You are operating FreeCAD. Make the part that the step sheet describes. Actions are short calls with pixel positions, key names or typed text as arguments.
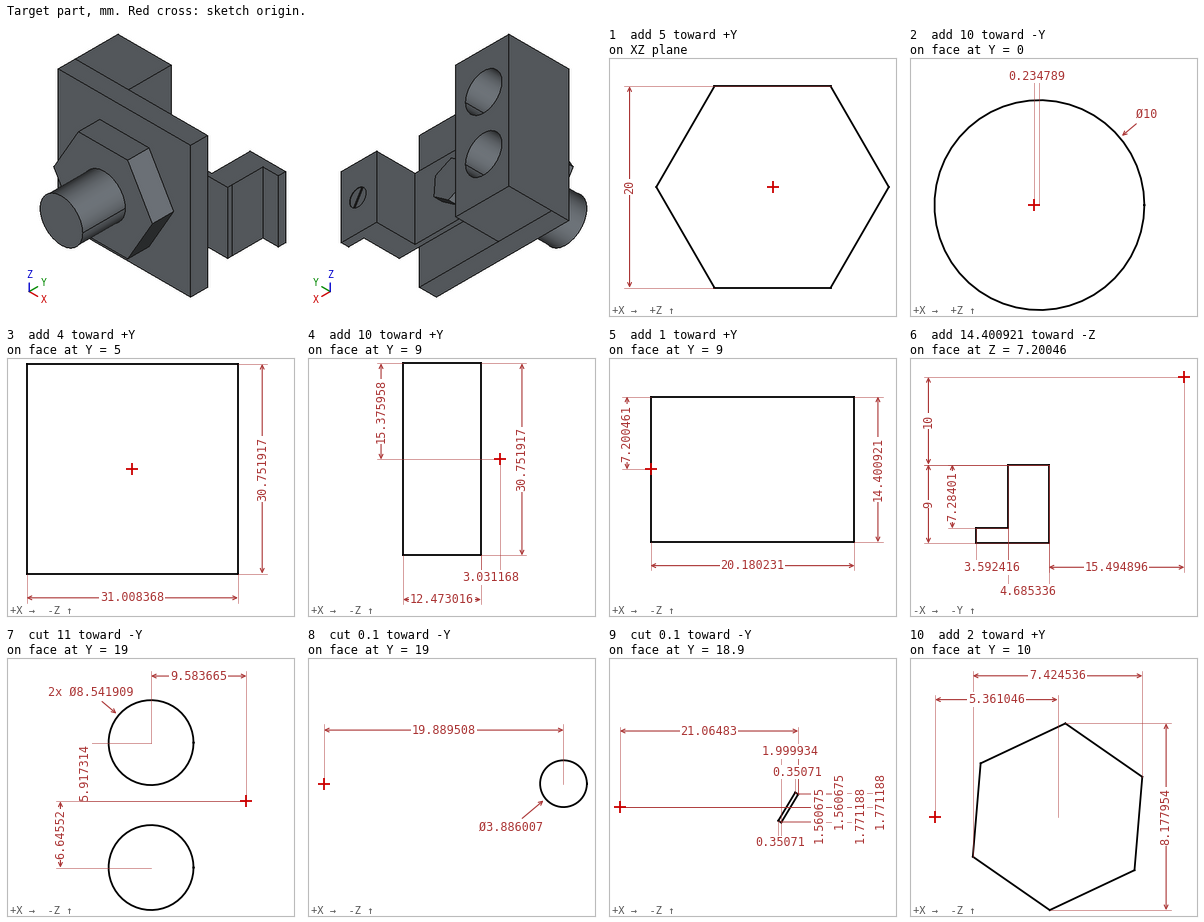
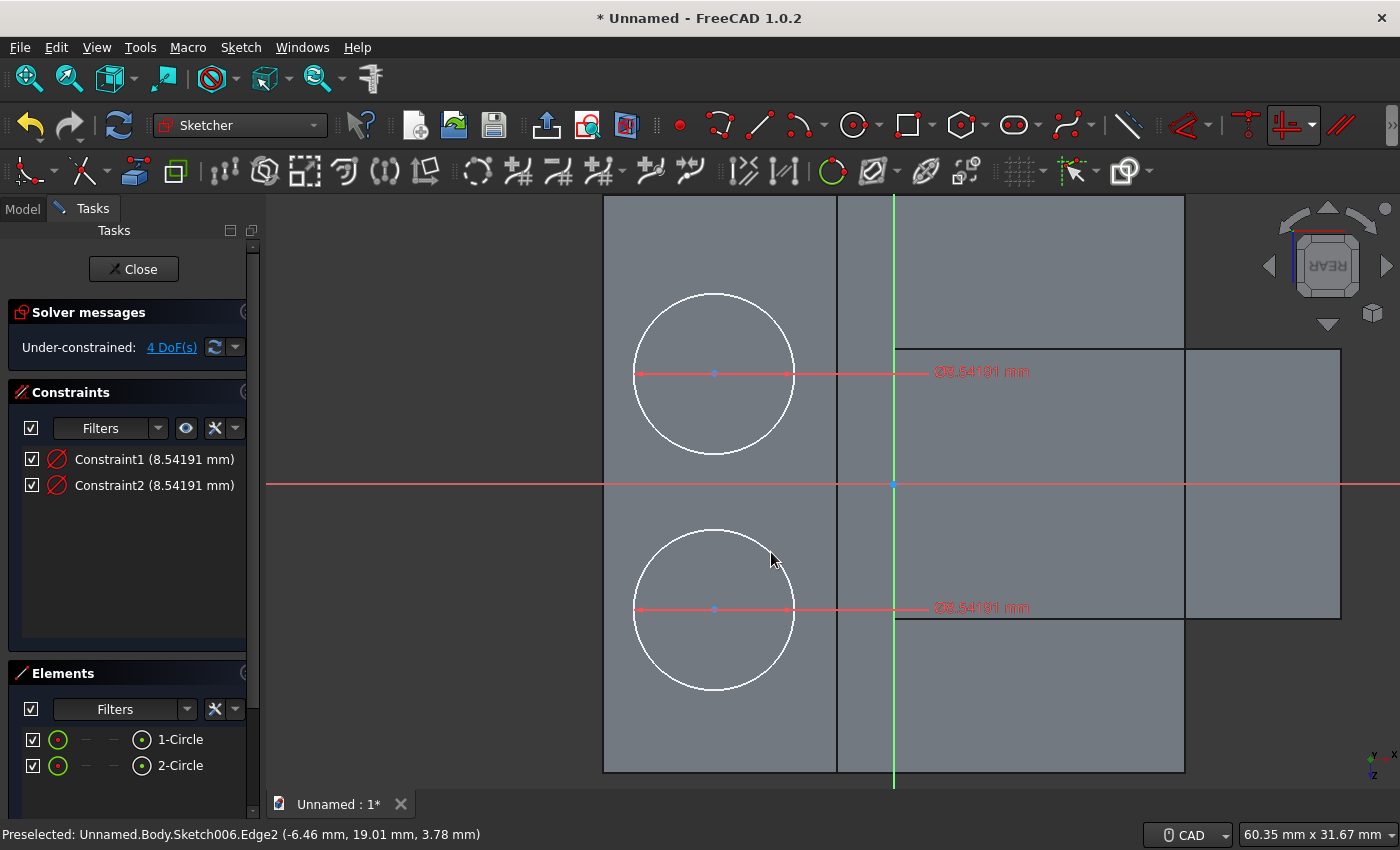
click(714, 374)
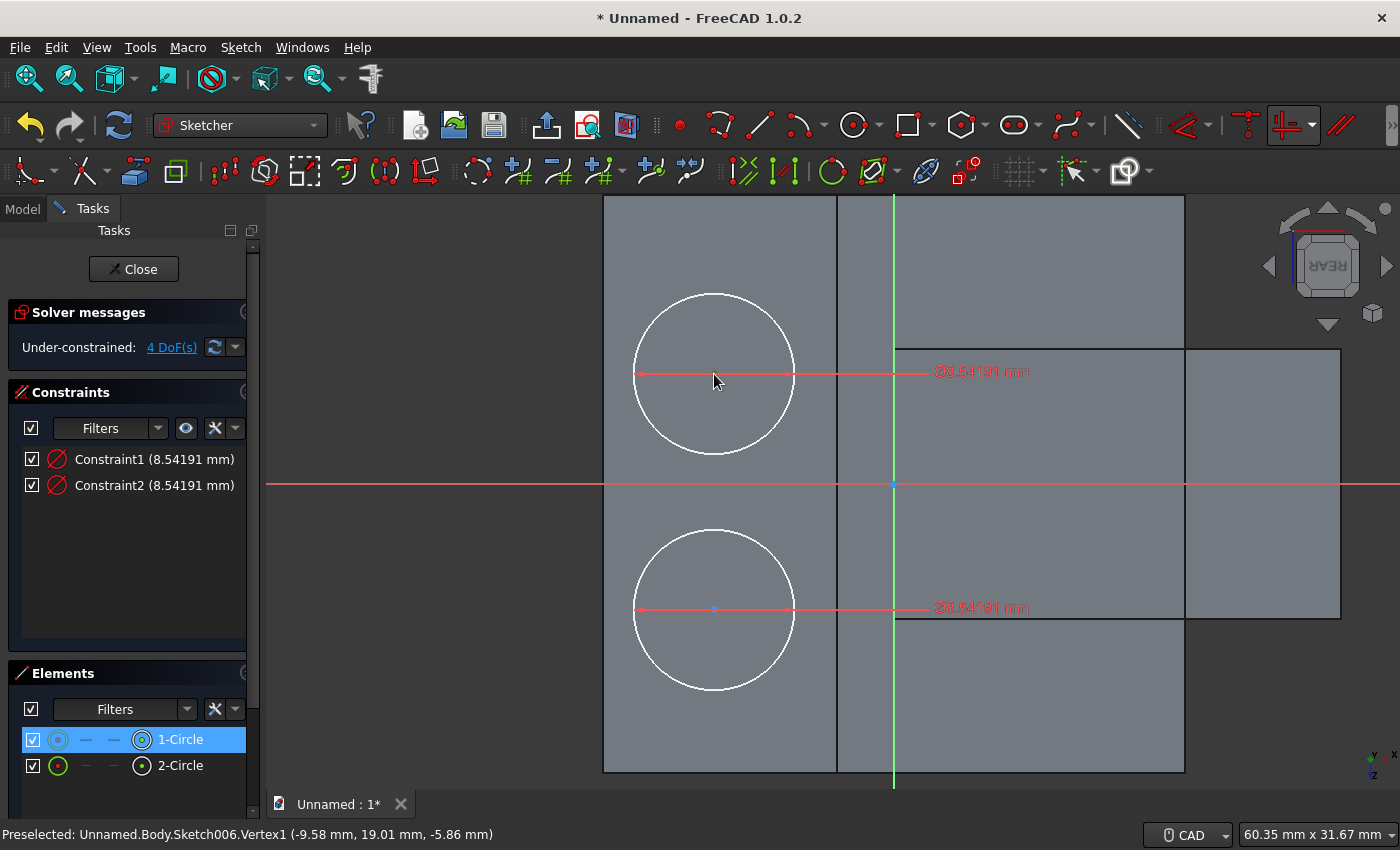
click(714, 610)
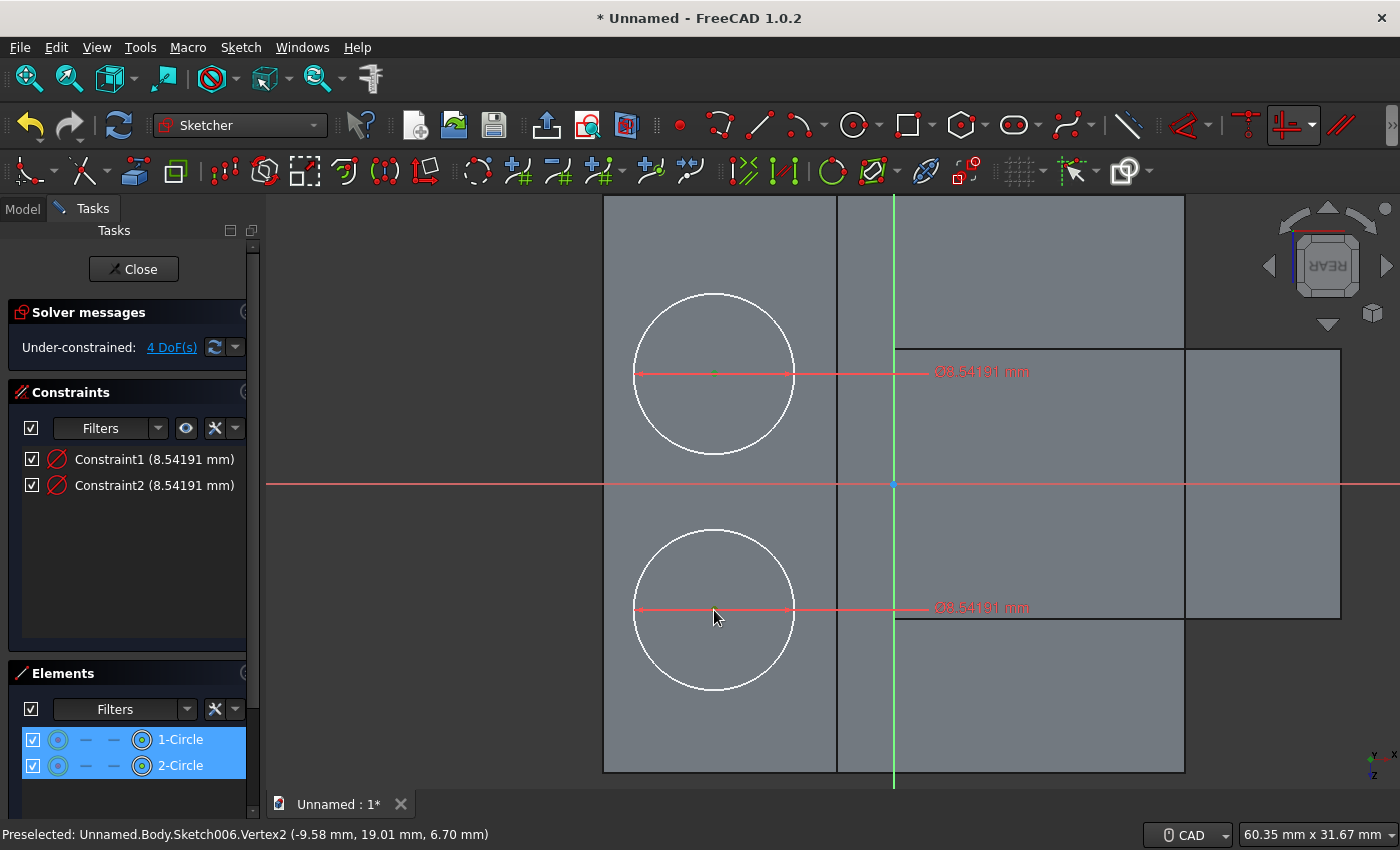
click(1314, 126)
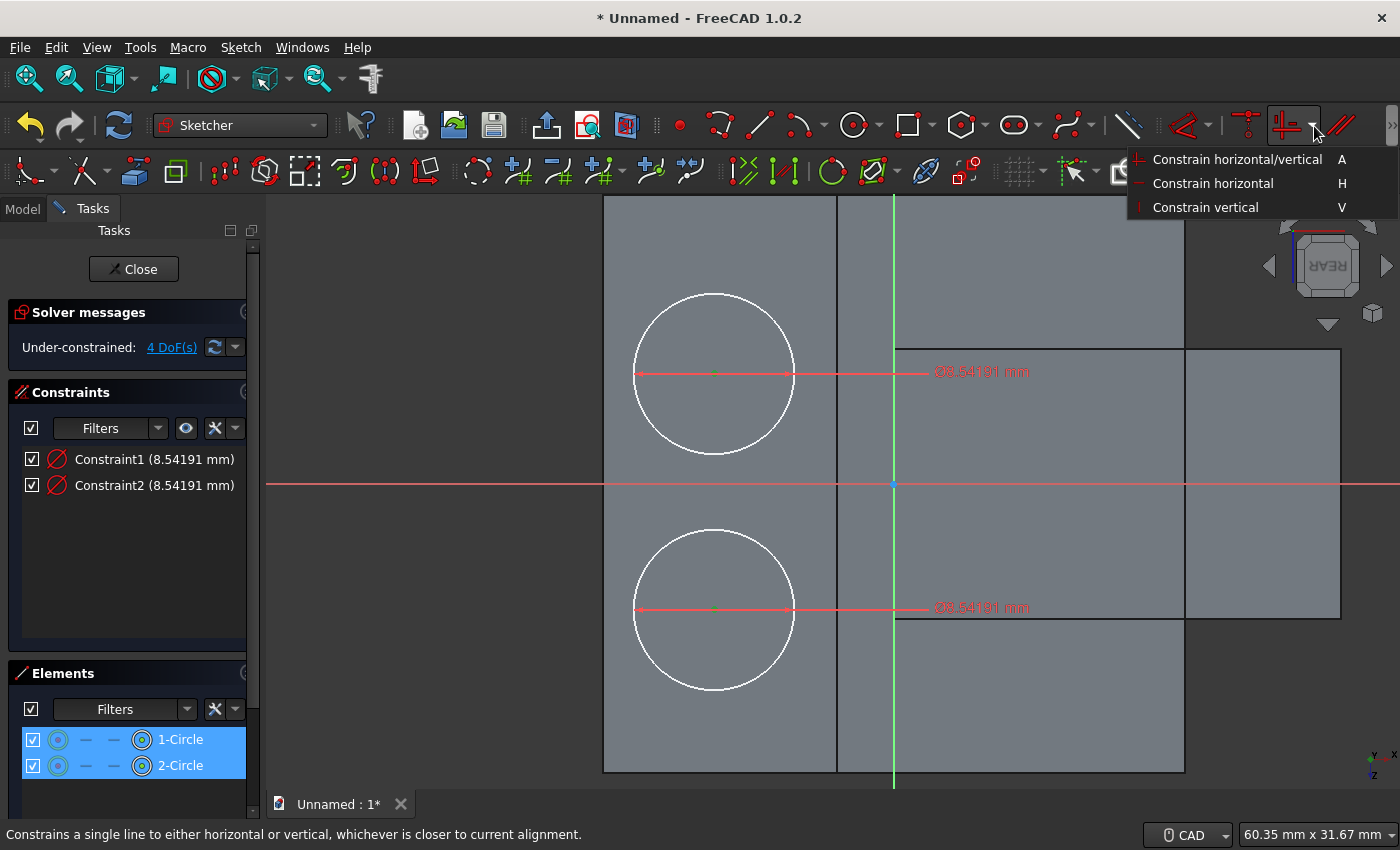
click(1263, 207)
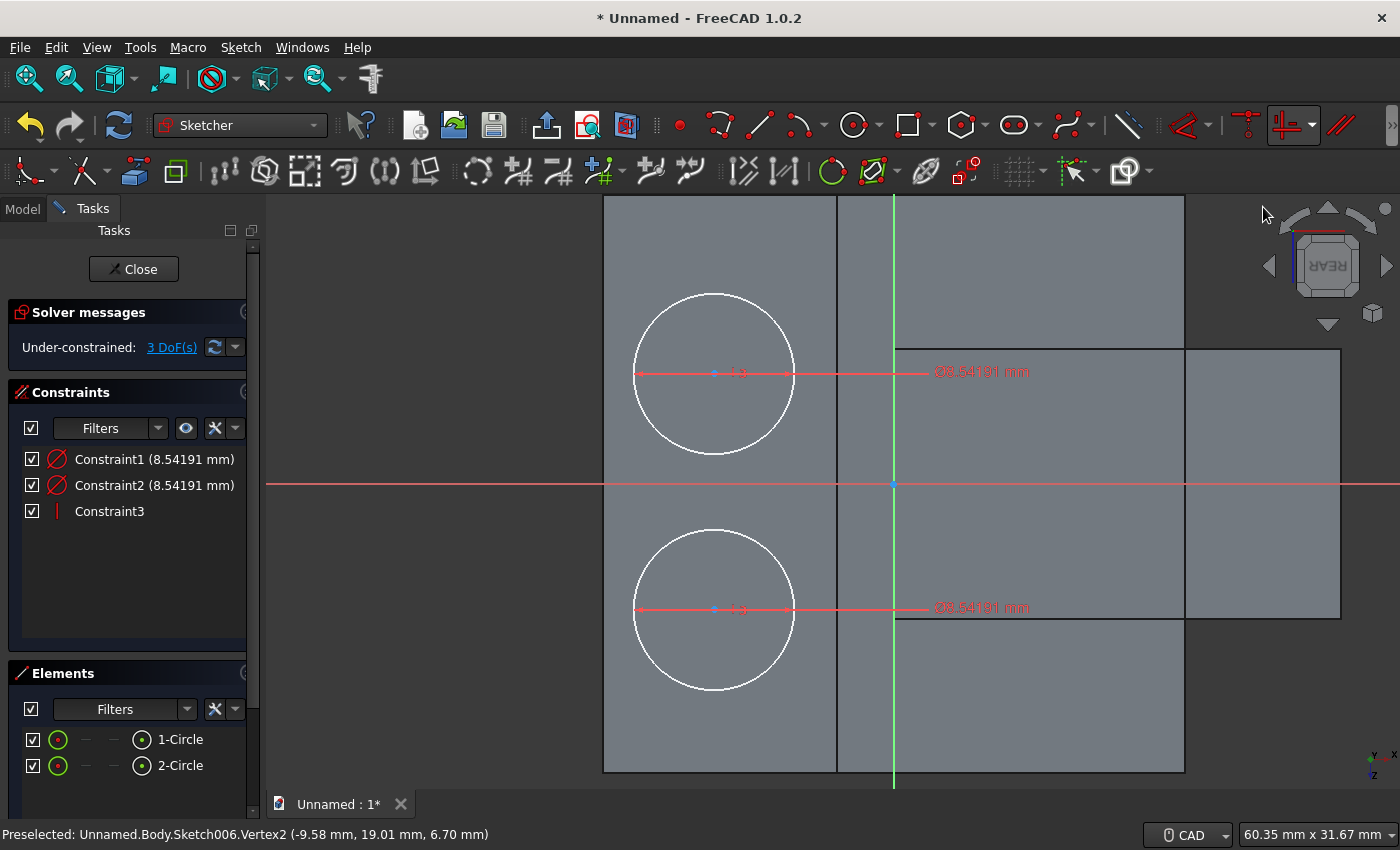
click(1184, 126)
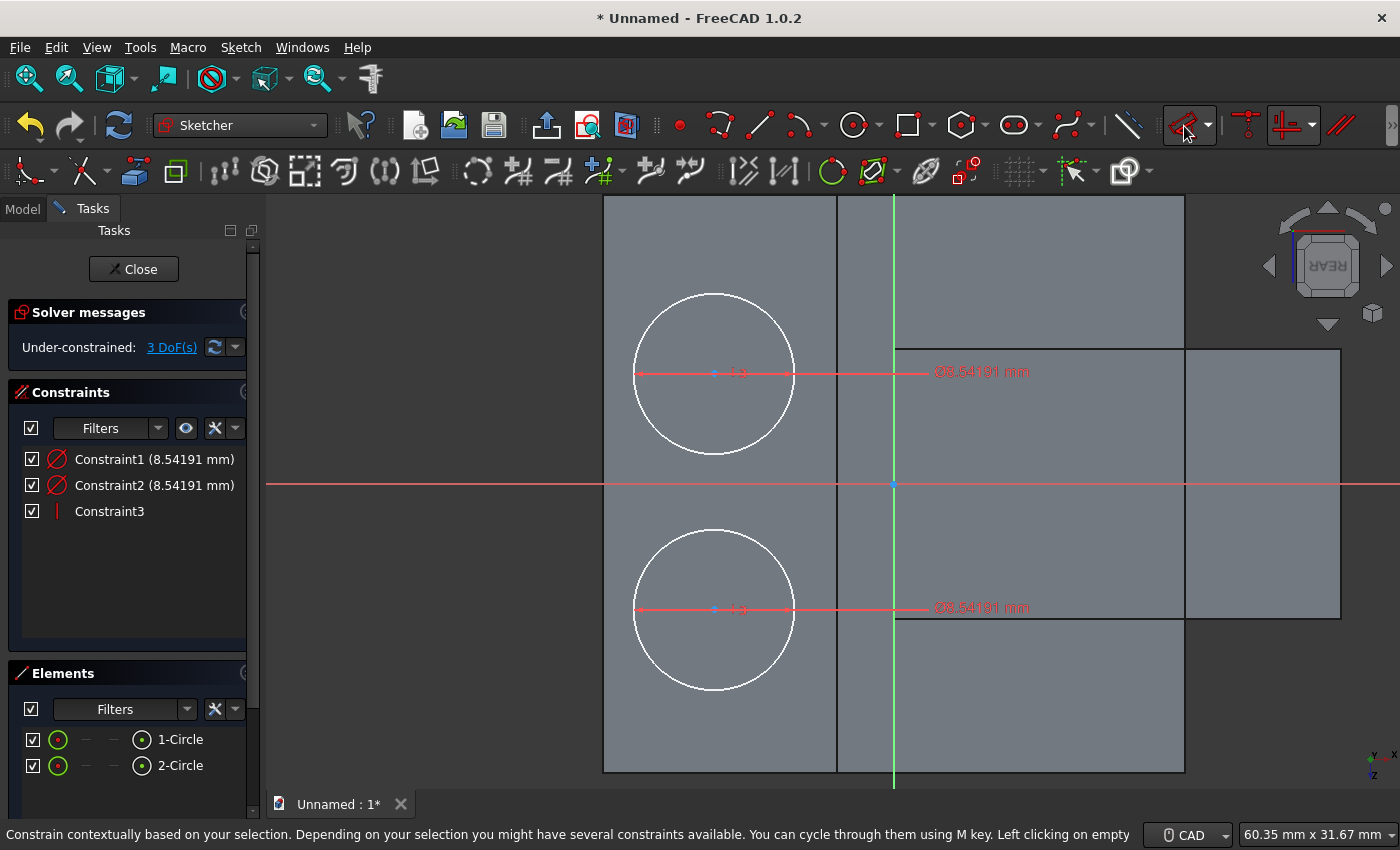
click(714, 610)
click(928, 547)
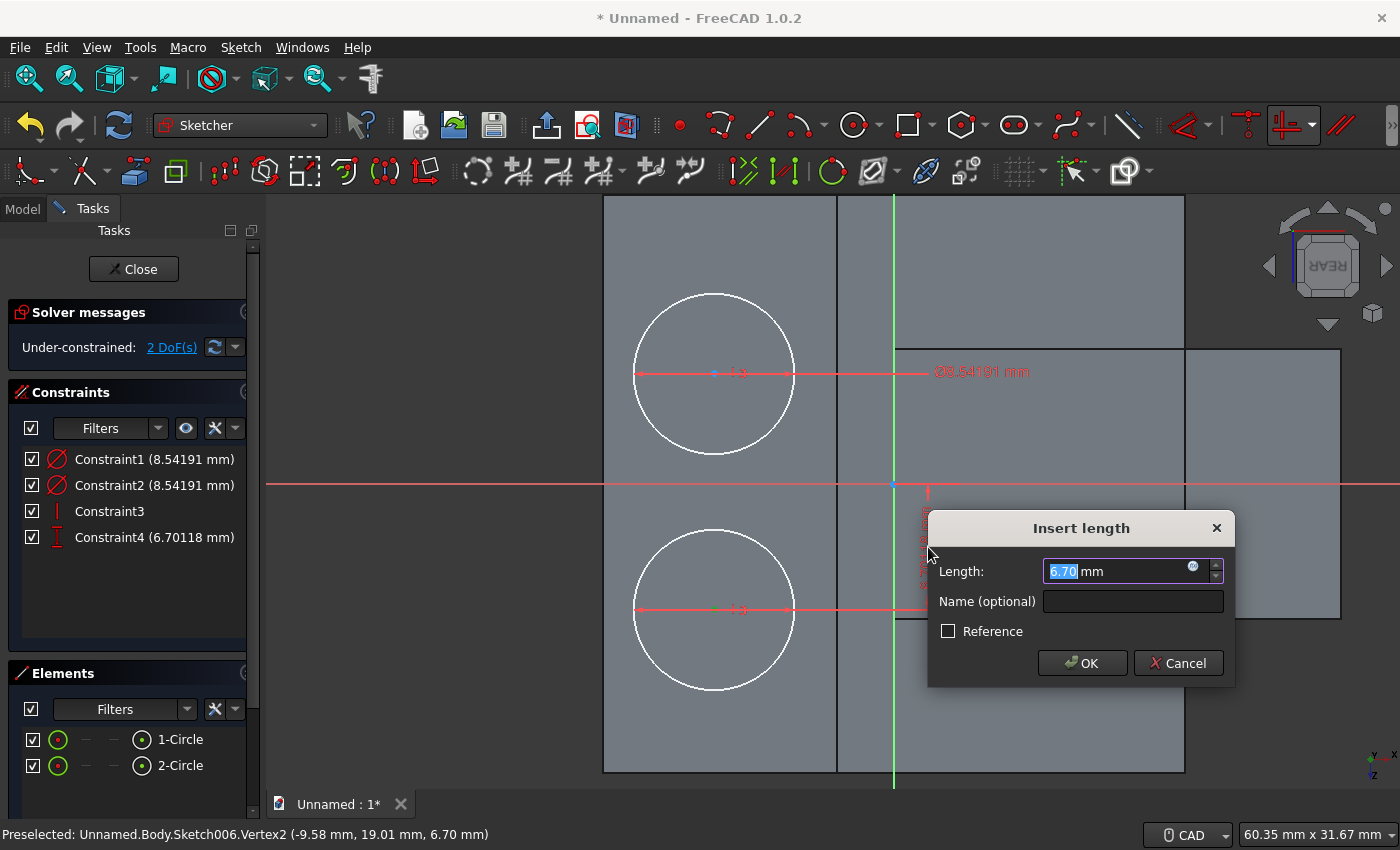
text(6.64552)
key(Return)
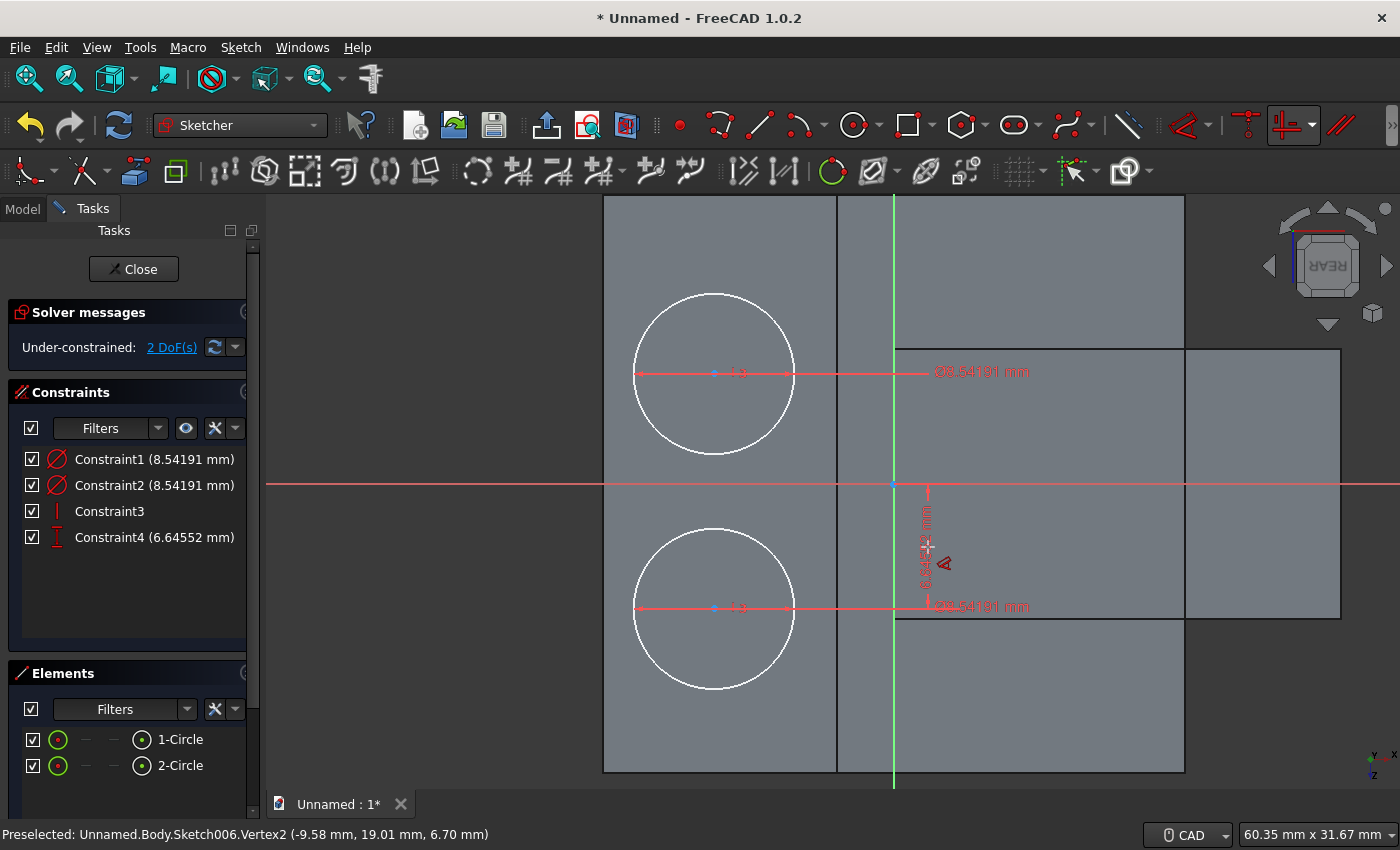
click(714, 374)
click(804, 340)